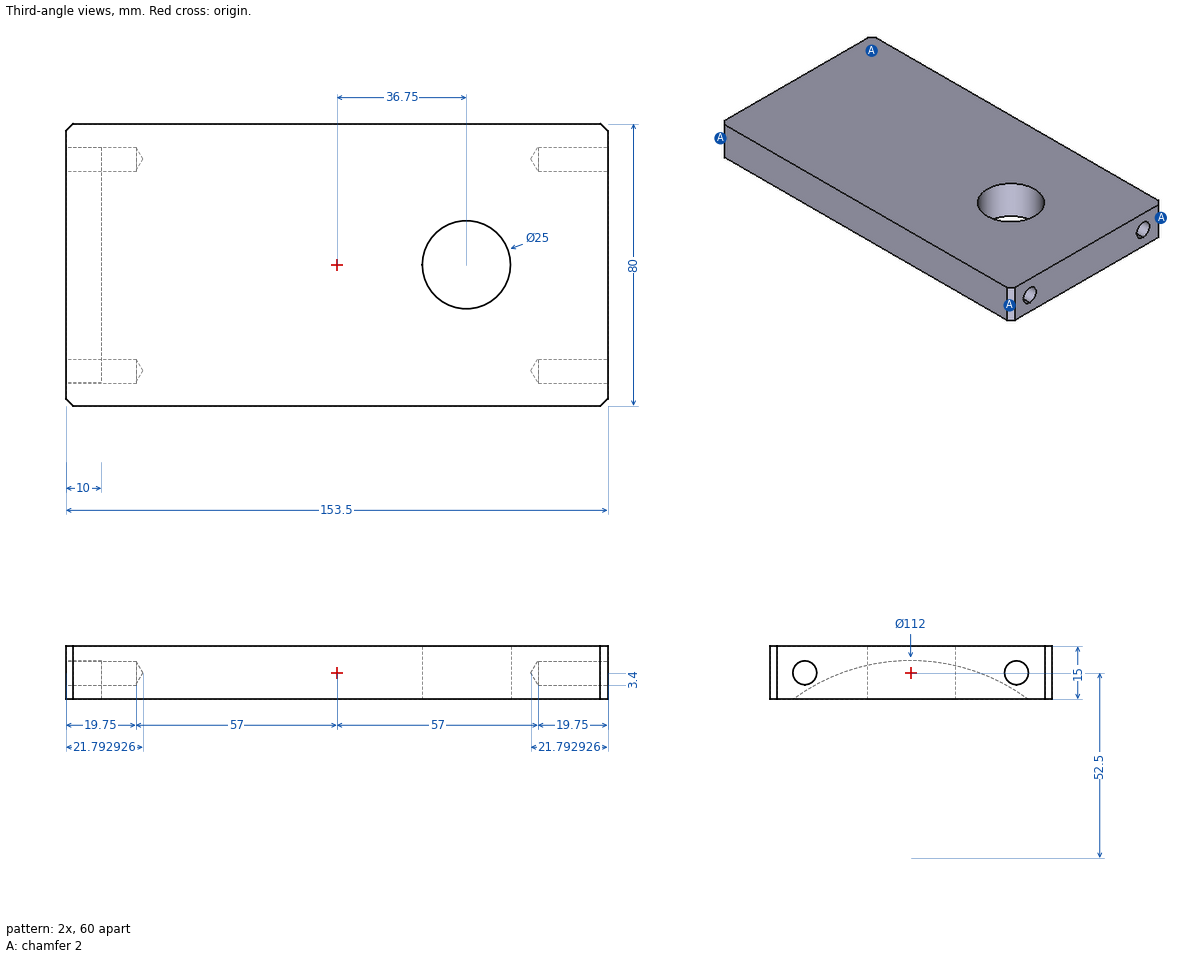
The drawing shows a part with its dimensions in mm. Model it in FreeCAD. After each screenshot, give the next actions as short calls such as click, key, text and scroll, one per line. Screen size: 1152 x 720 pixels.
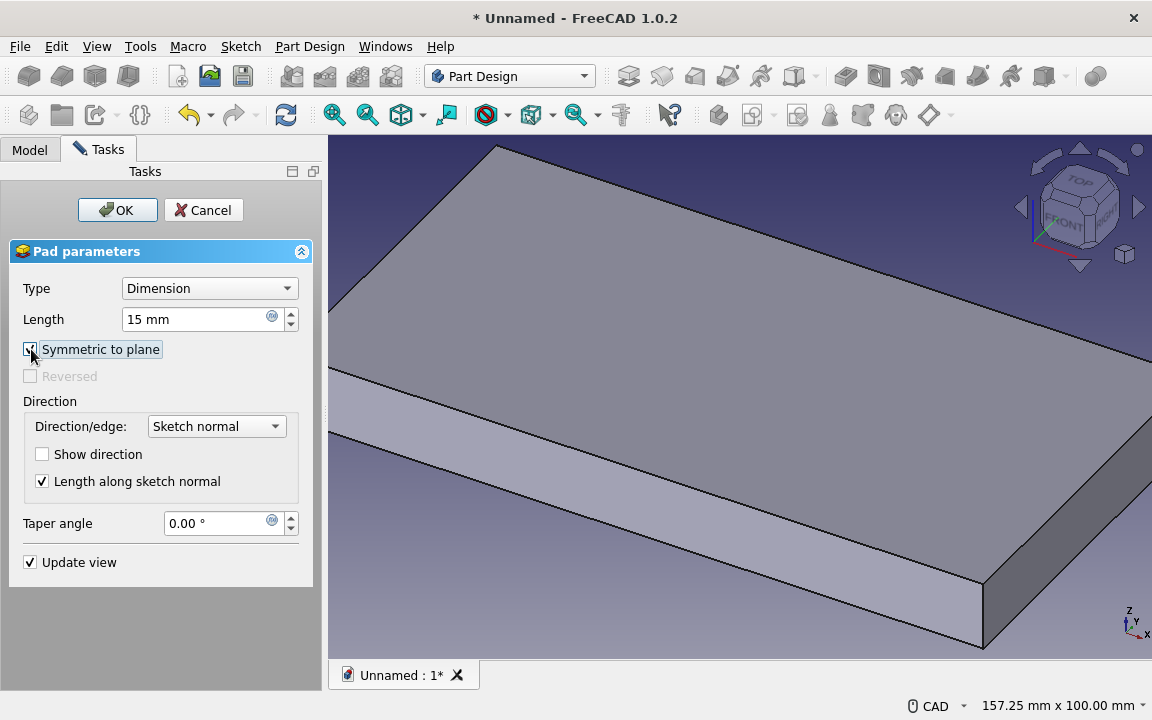
click(118, 210)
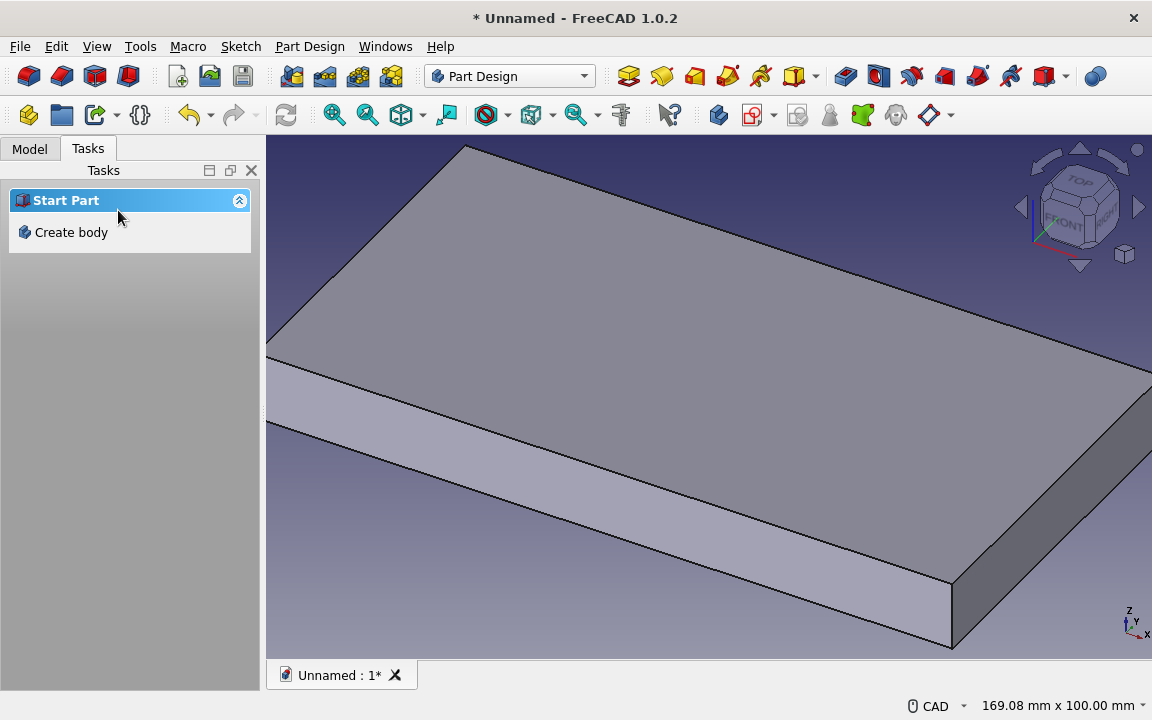
key(v)
key(f)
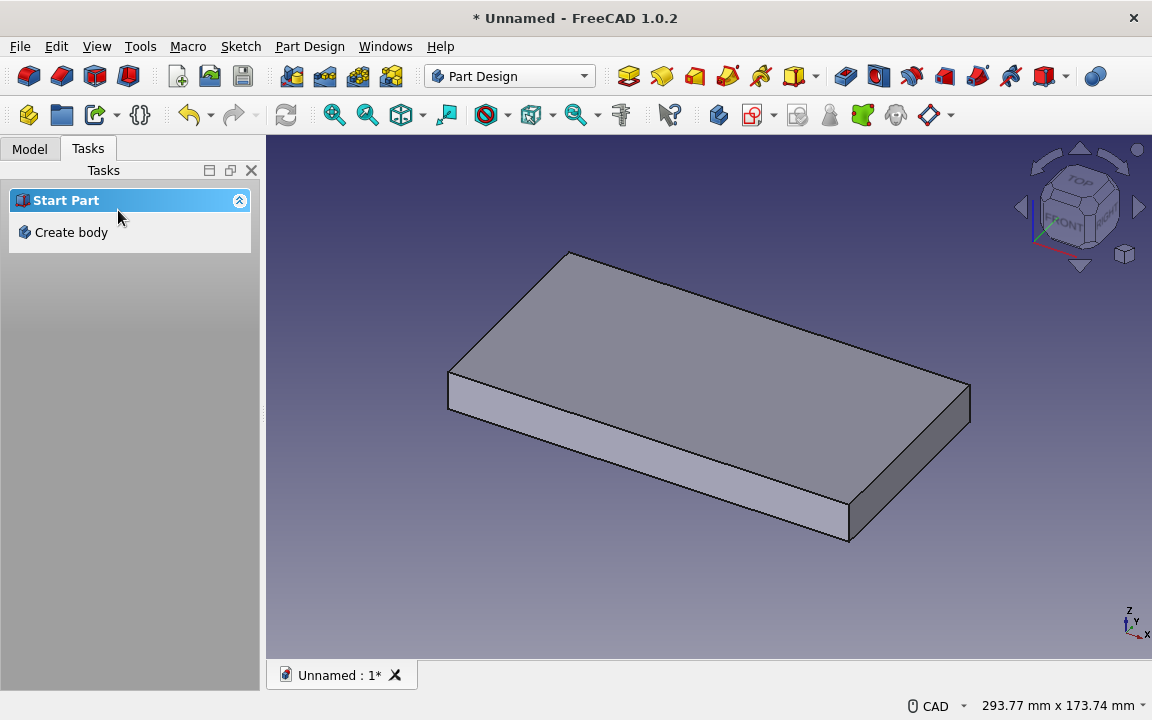
click(766, 396)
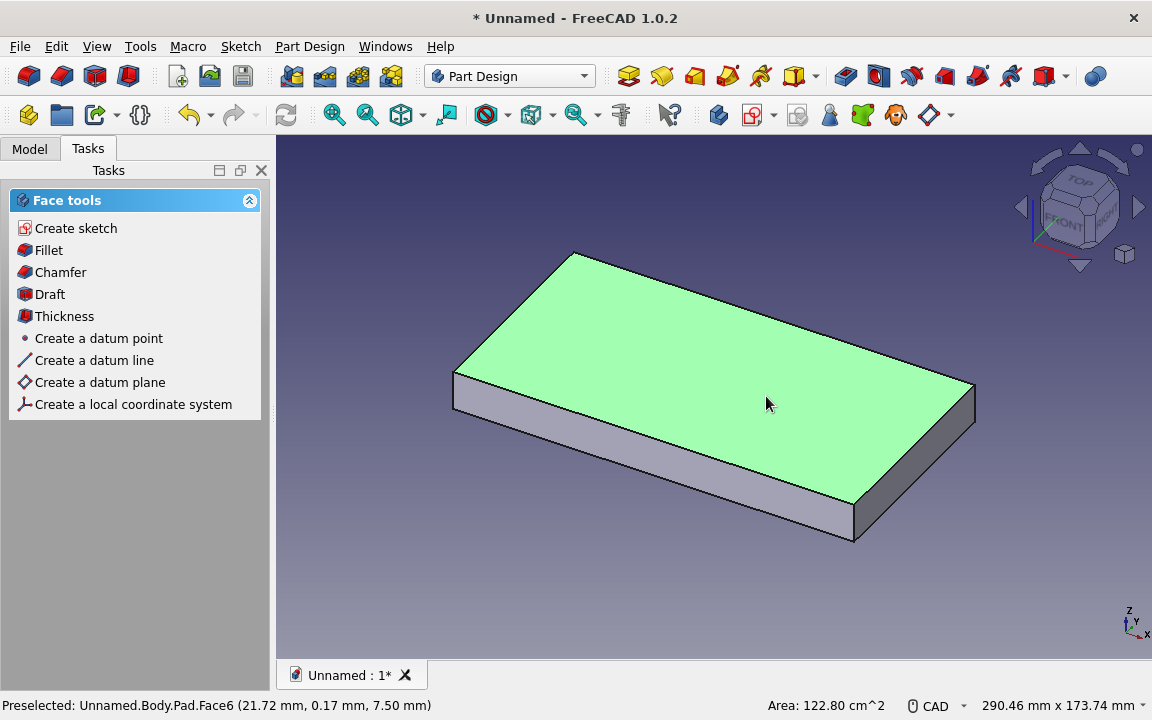
click(752, 116)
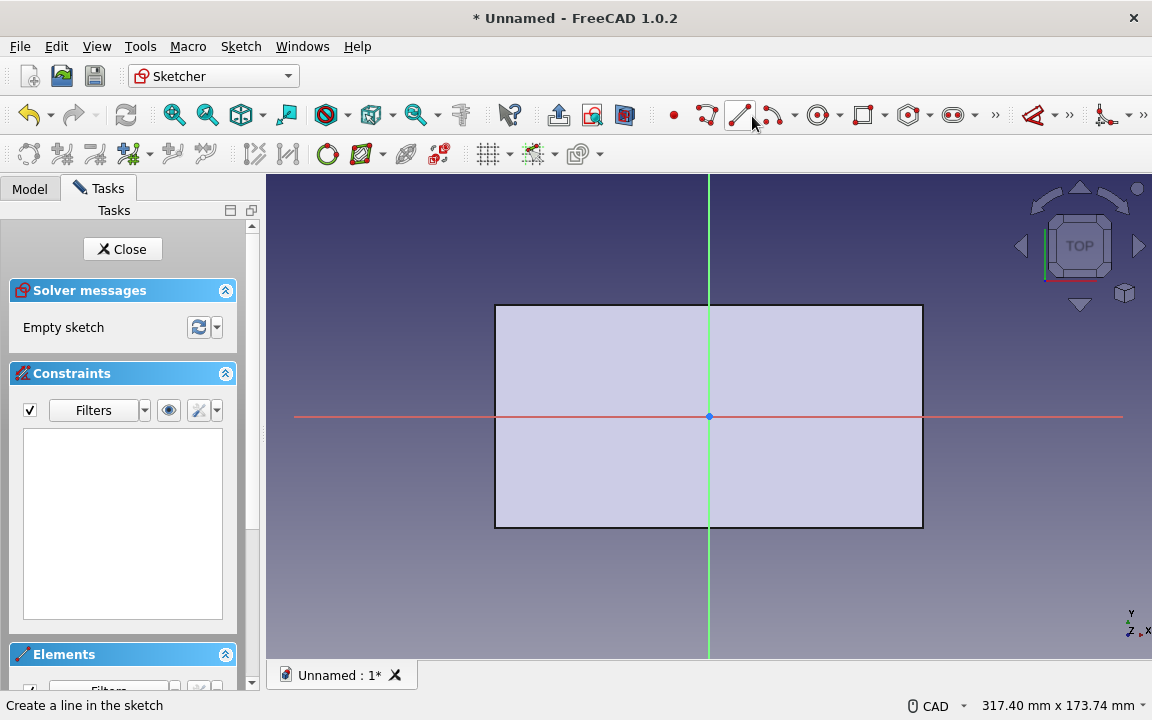
scroll(837, 416, up, 6)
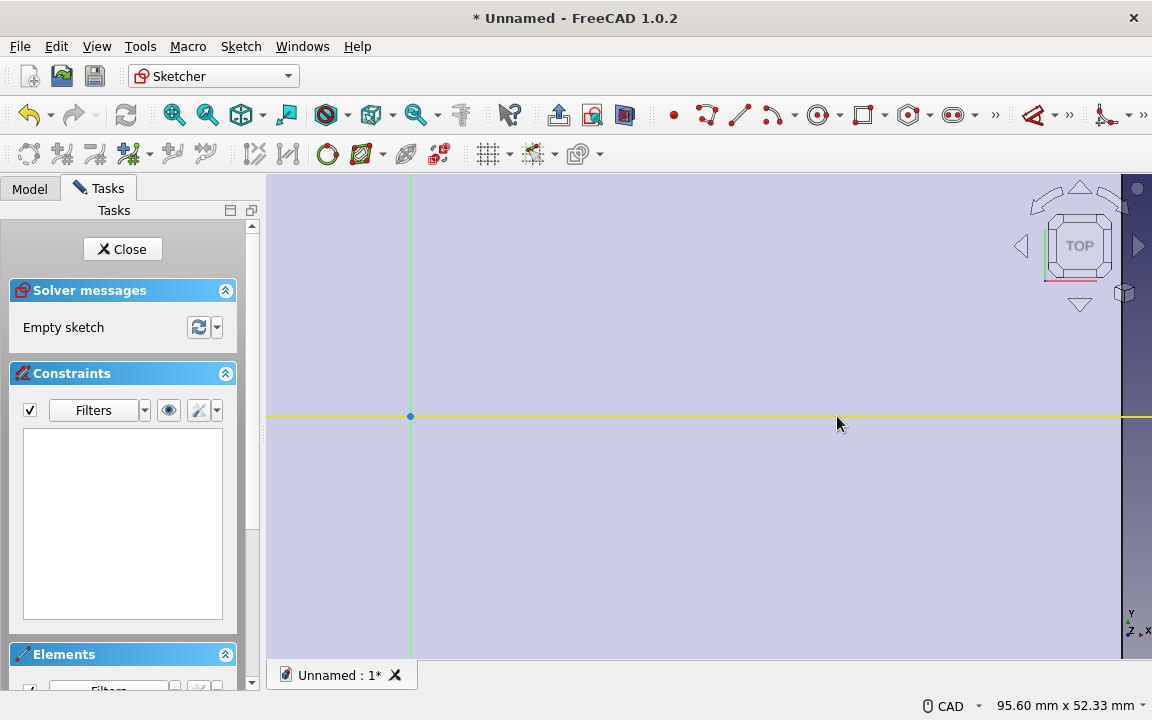
key(g)
key(c)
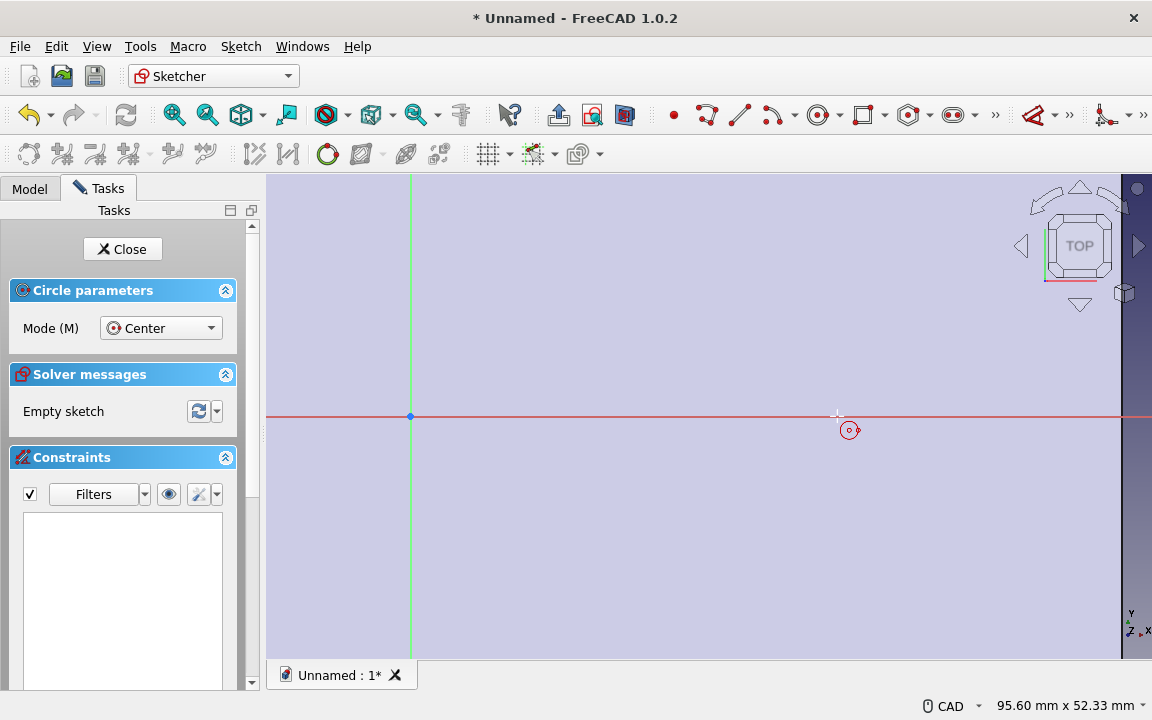
click(751, 416)
move(833, 335)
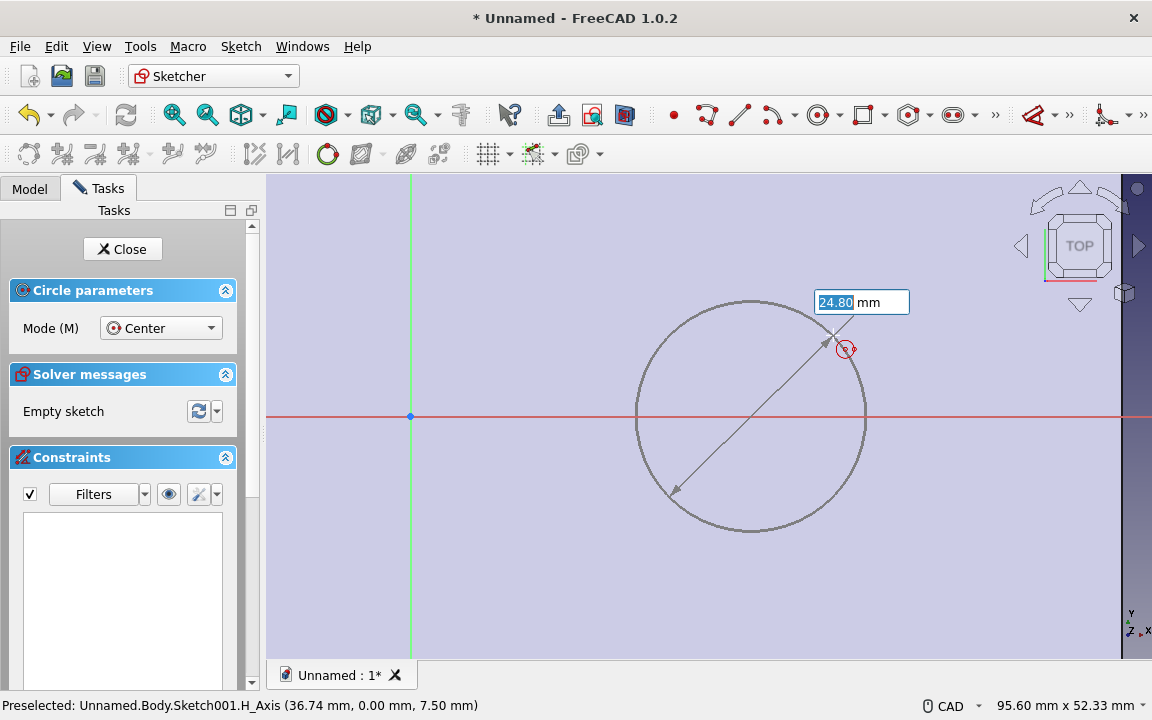
text(25)
key(Return)
key(Escape)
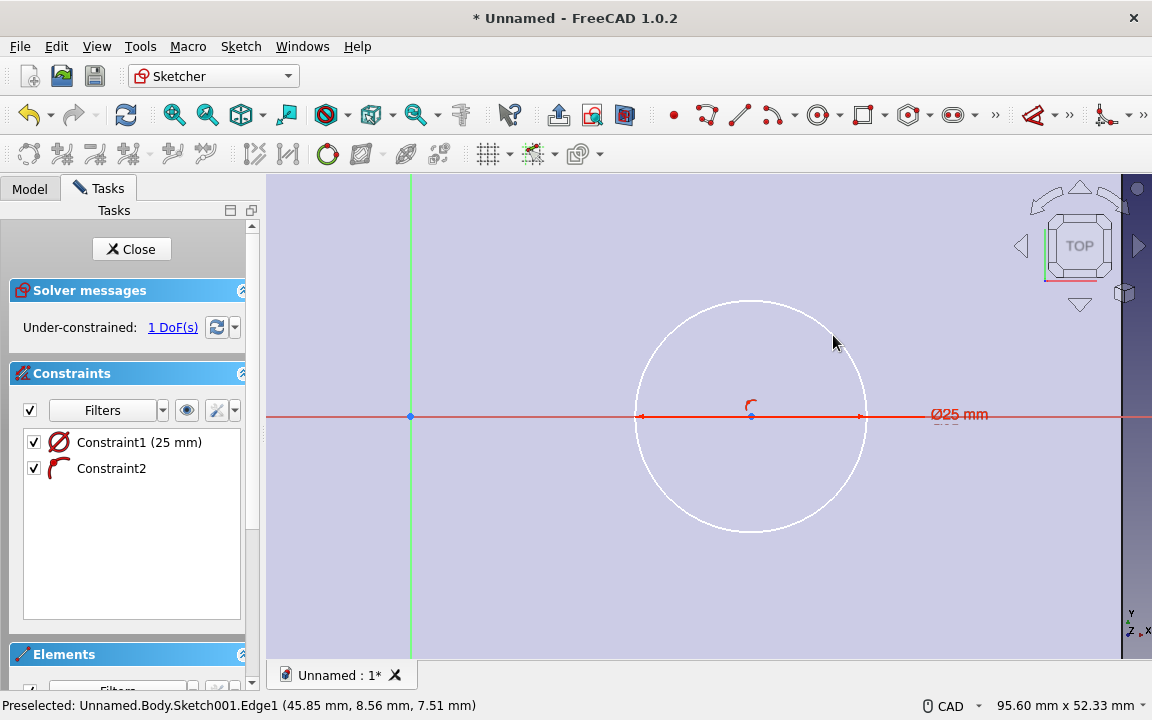
click(1032, 116)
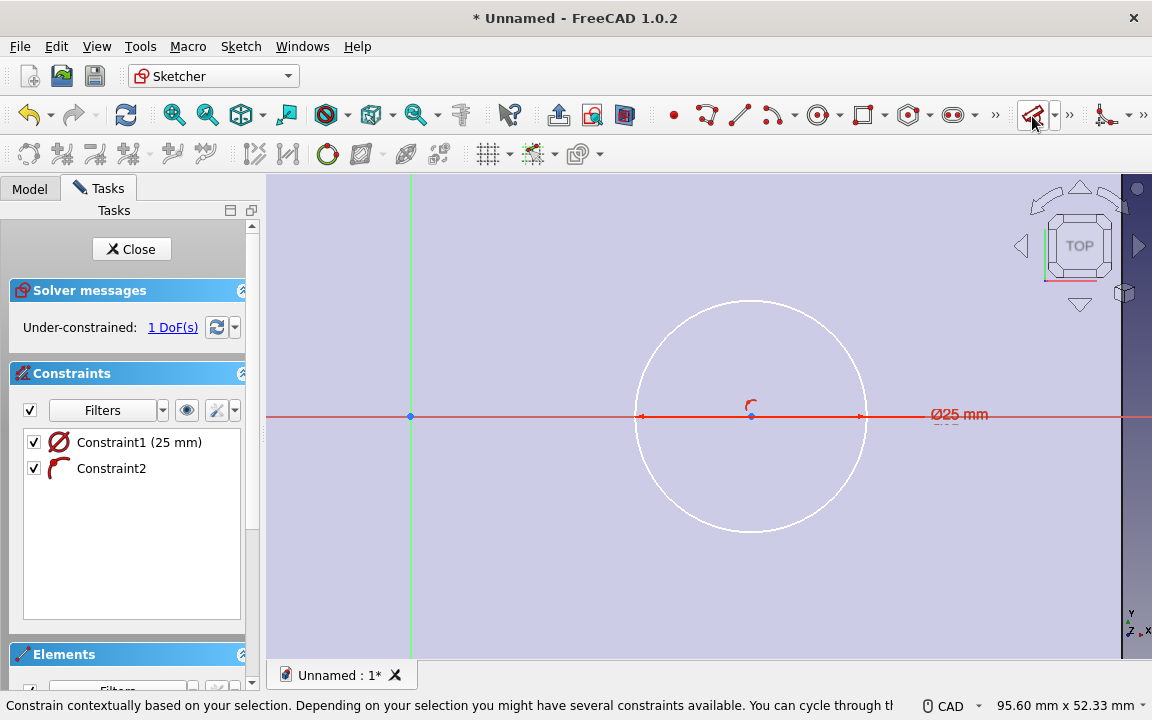
click(751, 416)
click(581, 450)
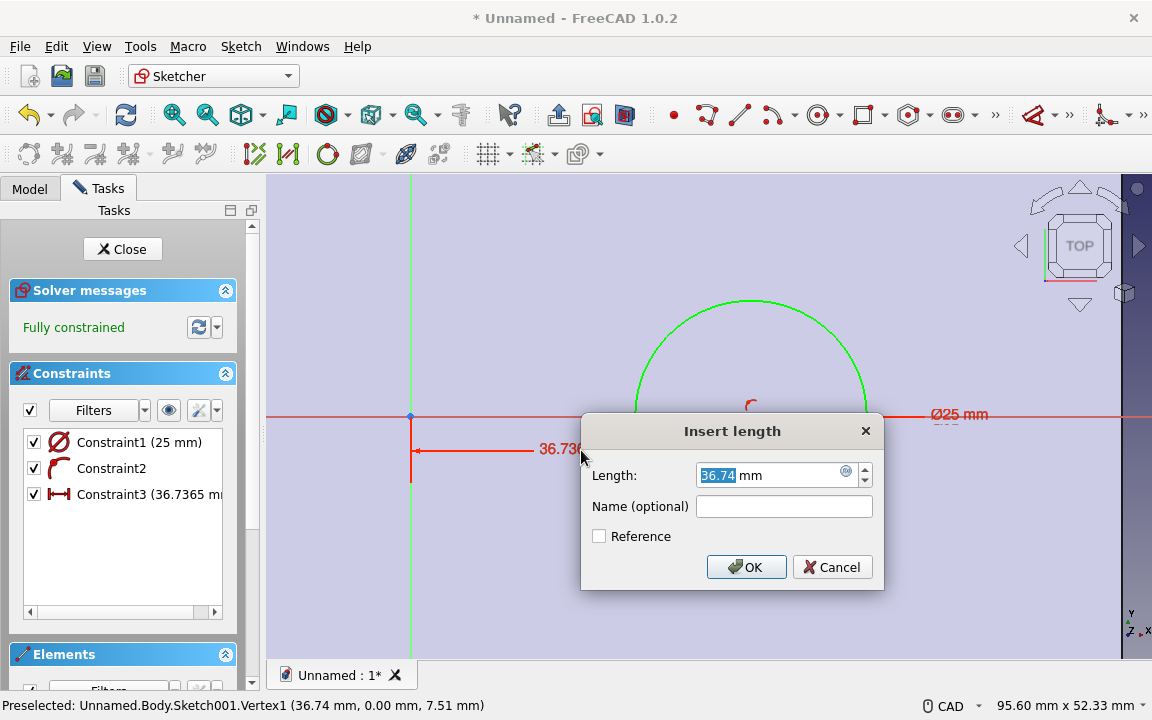
text(36.75)
key(Return)
key(Escape)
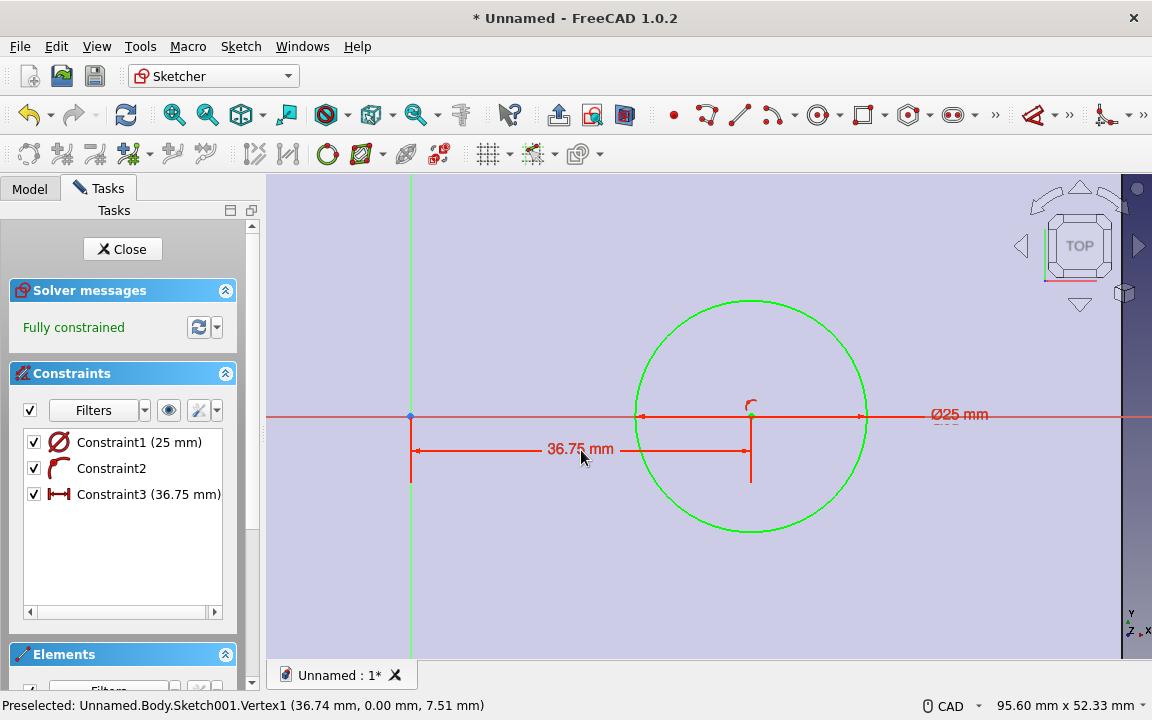
click(123, 249)